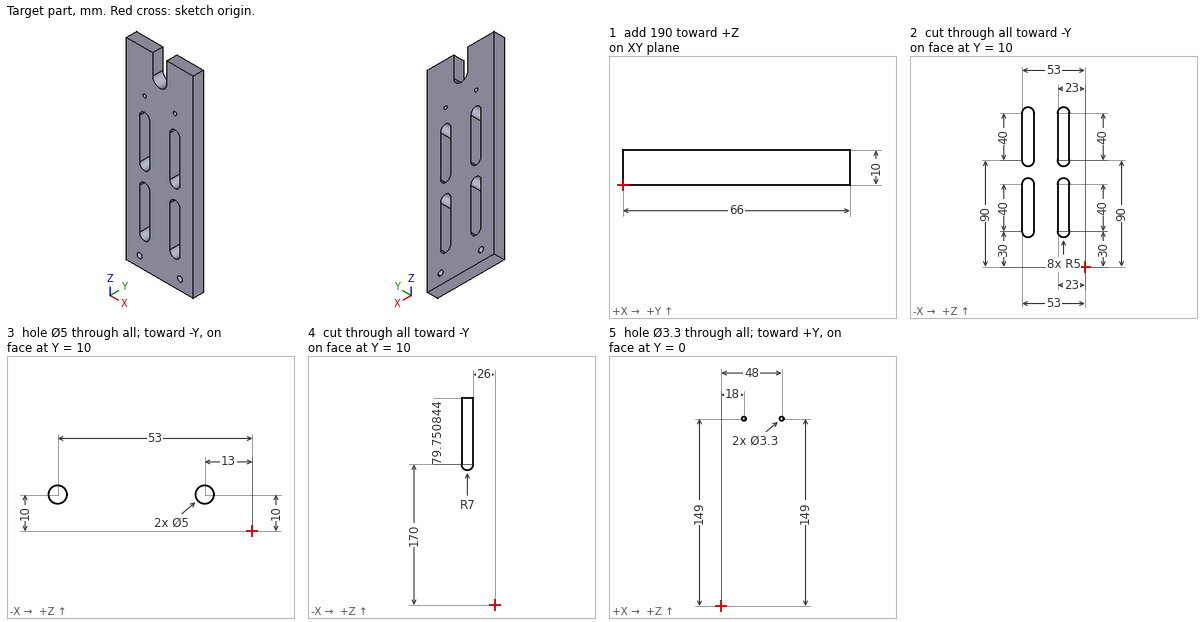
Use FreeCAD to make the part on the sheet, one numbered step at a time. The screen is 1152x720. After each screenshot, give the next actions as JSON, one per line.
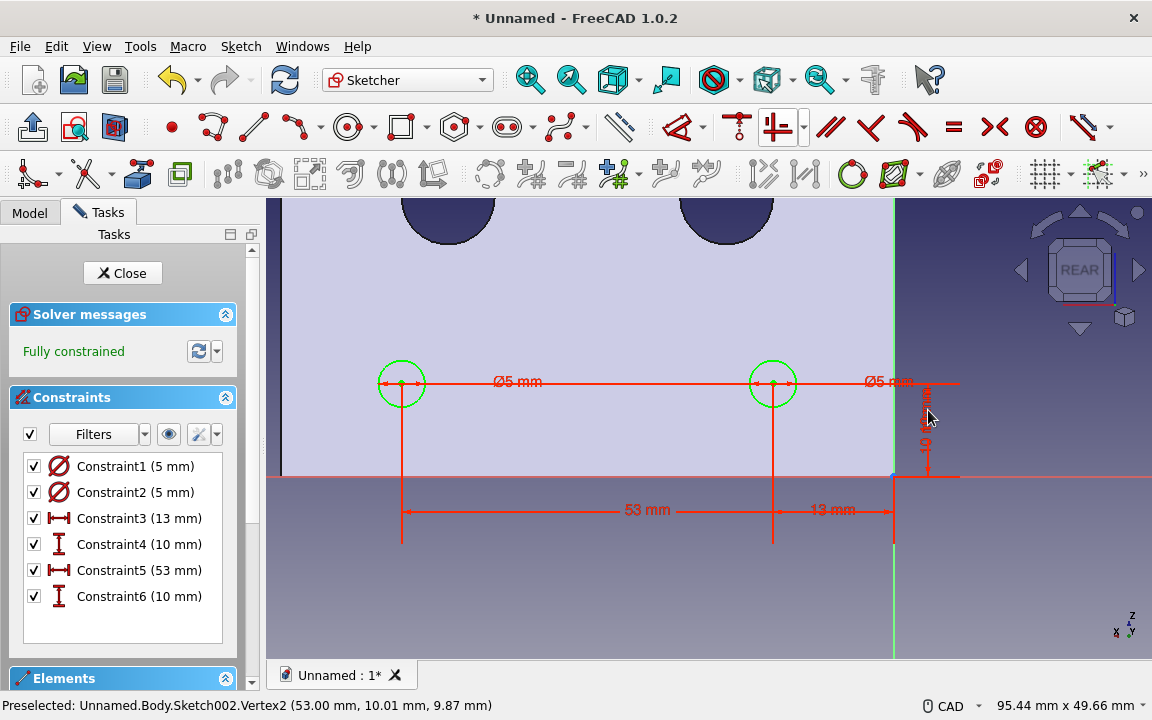
{"action": "left_click", "coordinate": [123, 273]}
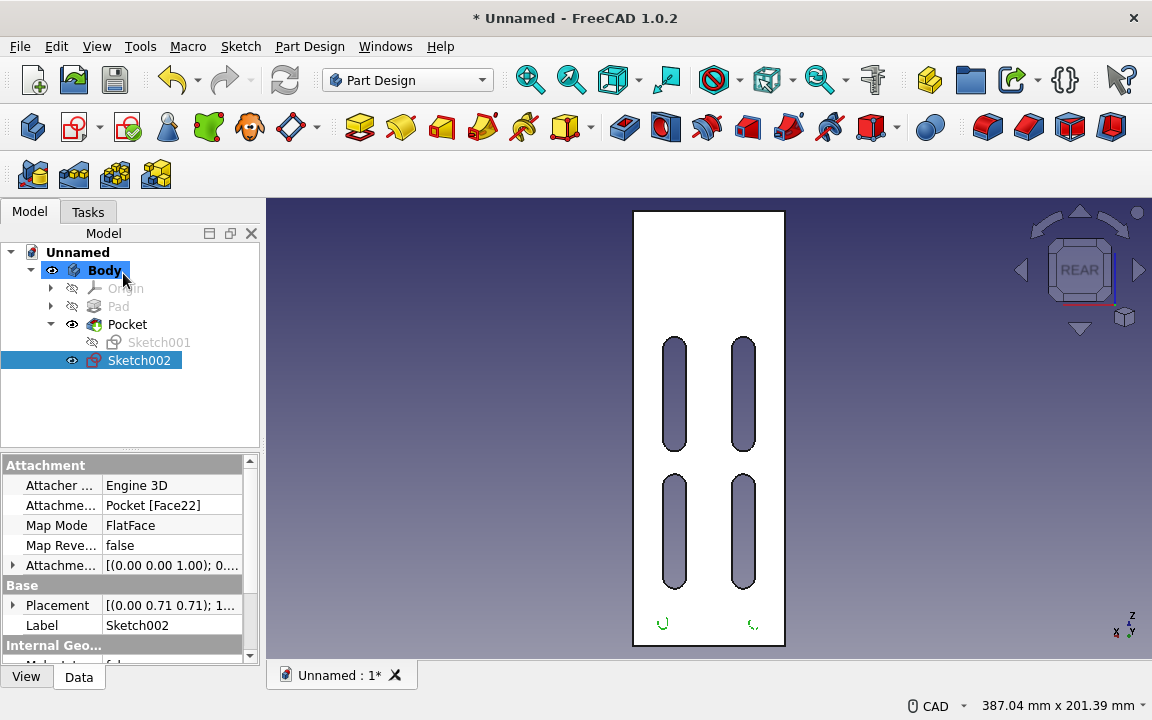
{"action": "left_click", "coordinate": [666, 128]}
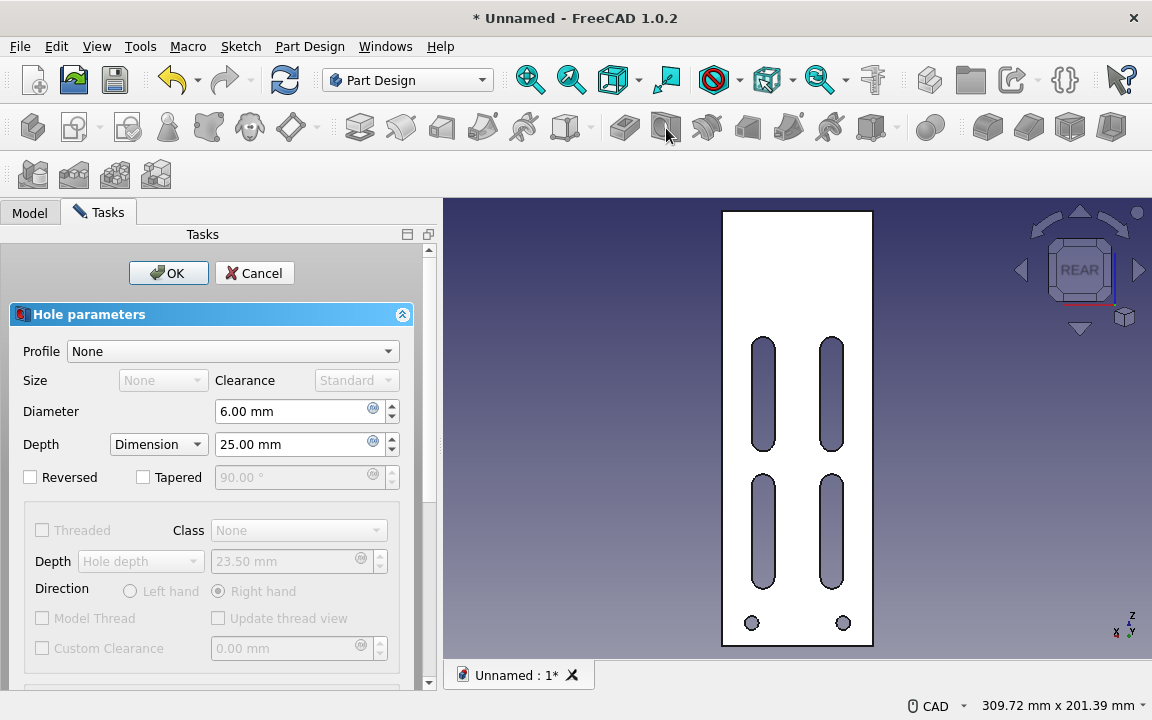
{"action": "triple_click", "coordinate": [300, 412]}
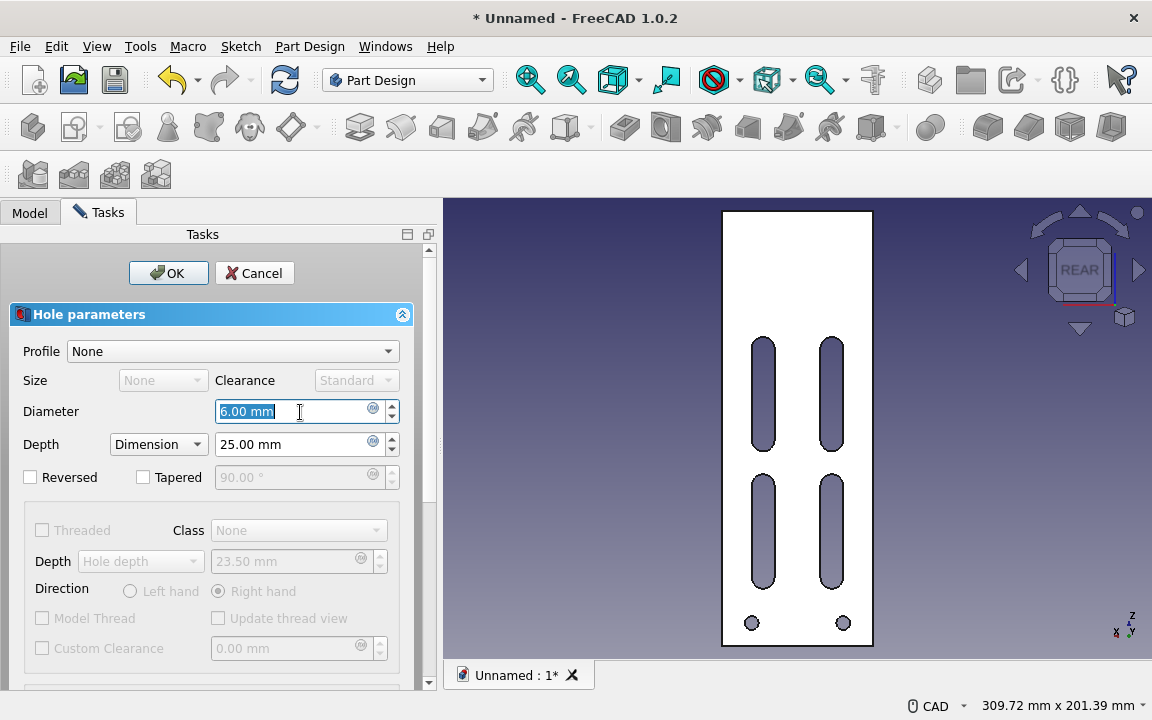
{"action": "type", "text": "5"}
{"action": "key", "text": "Tab"}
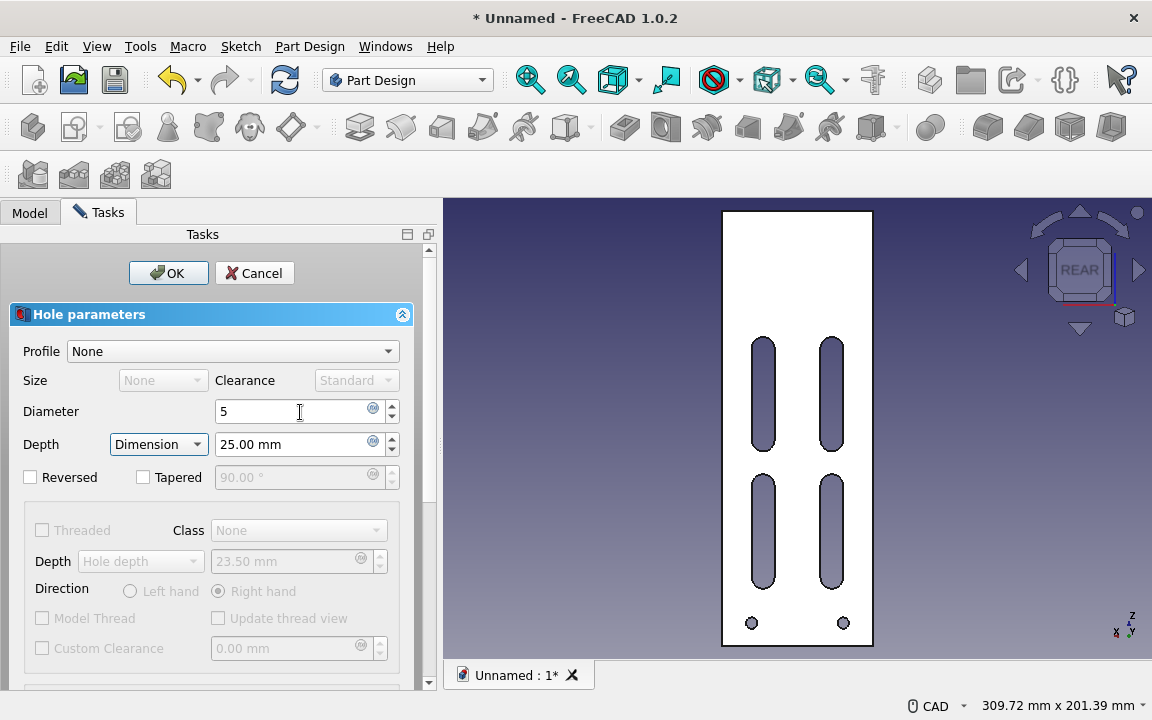
{"action": "left_click", "coordinate": [160, 444]}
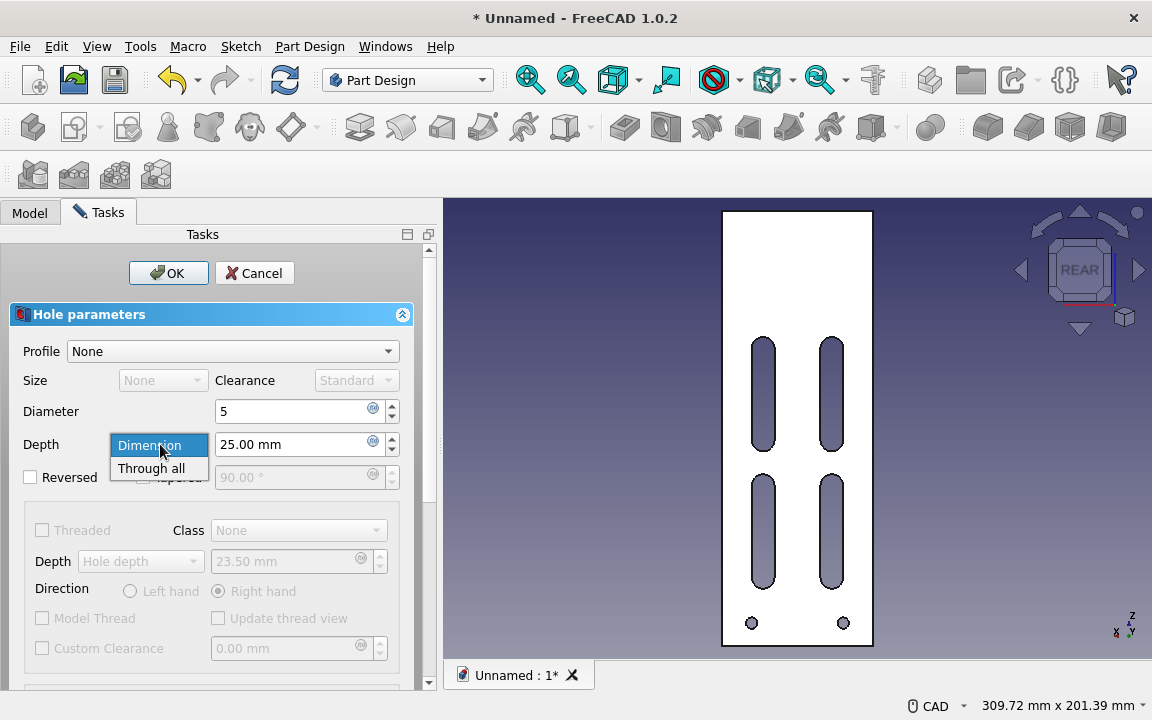
{"action": "left_click", "coordinate": [158, 468]}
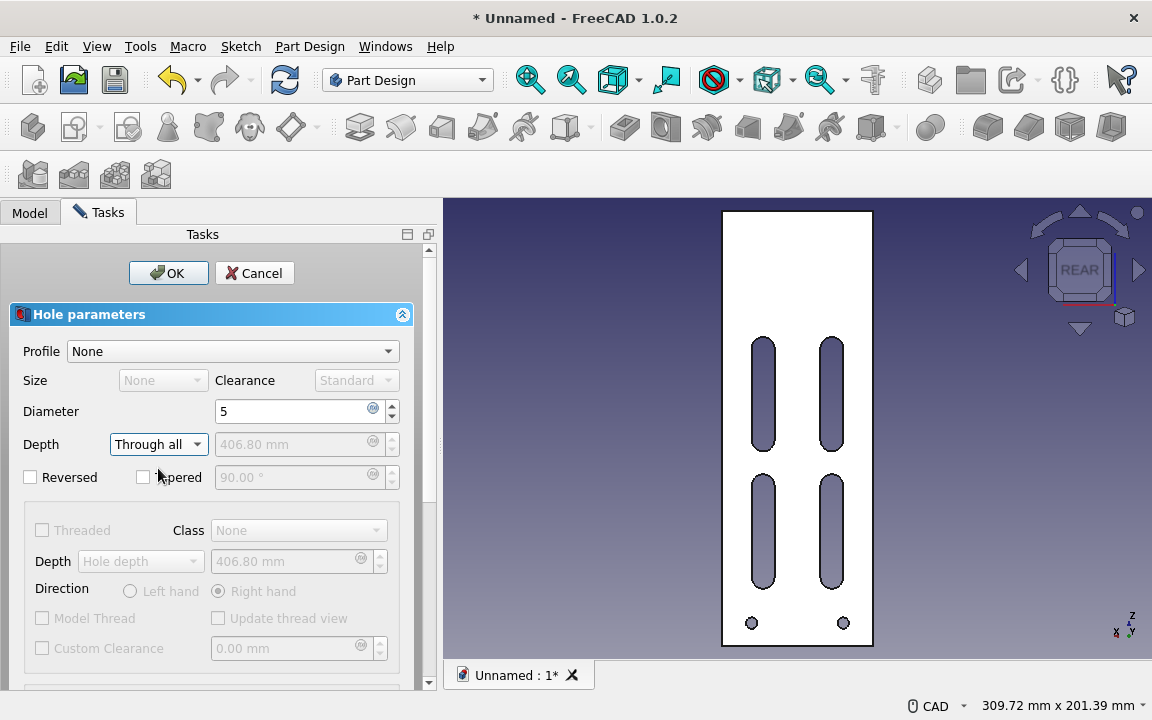
{"action": "left_click", "coordinate": [169, 273]}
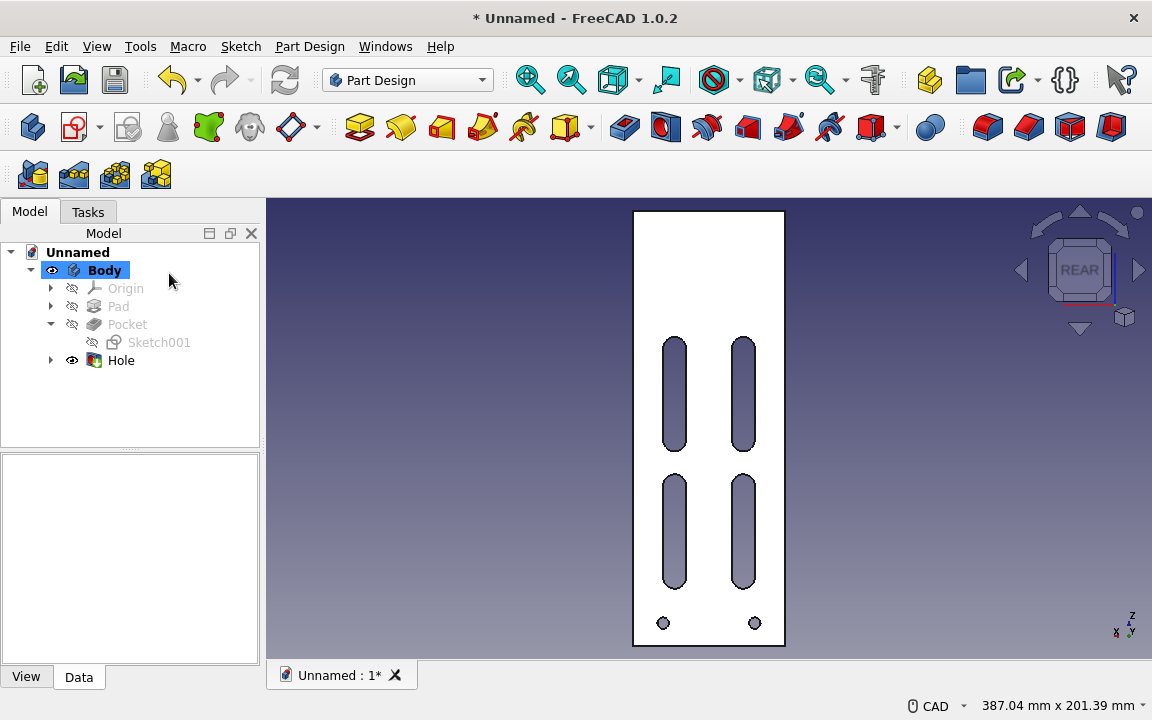
{"action": "left_click", "coordinate": [709, 303]}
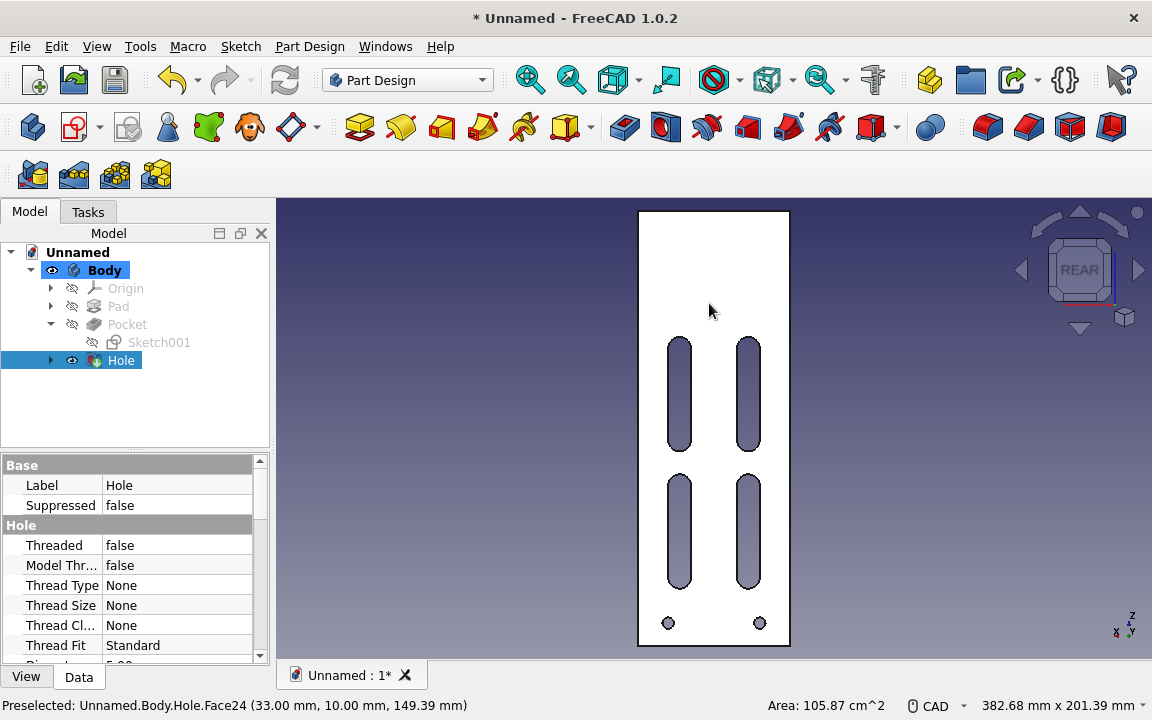
{"action": "left_click", "coordinate": [74, 128]}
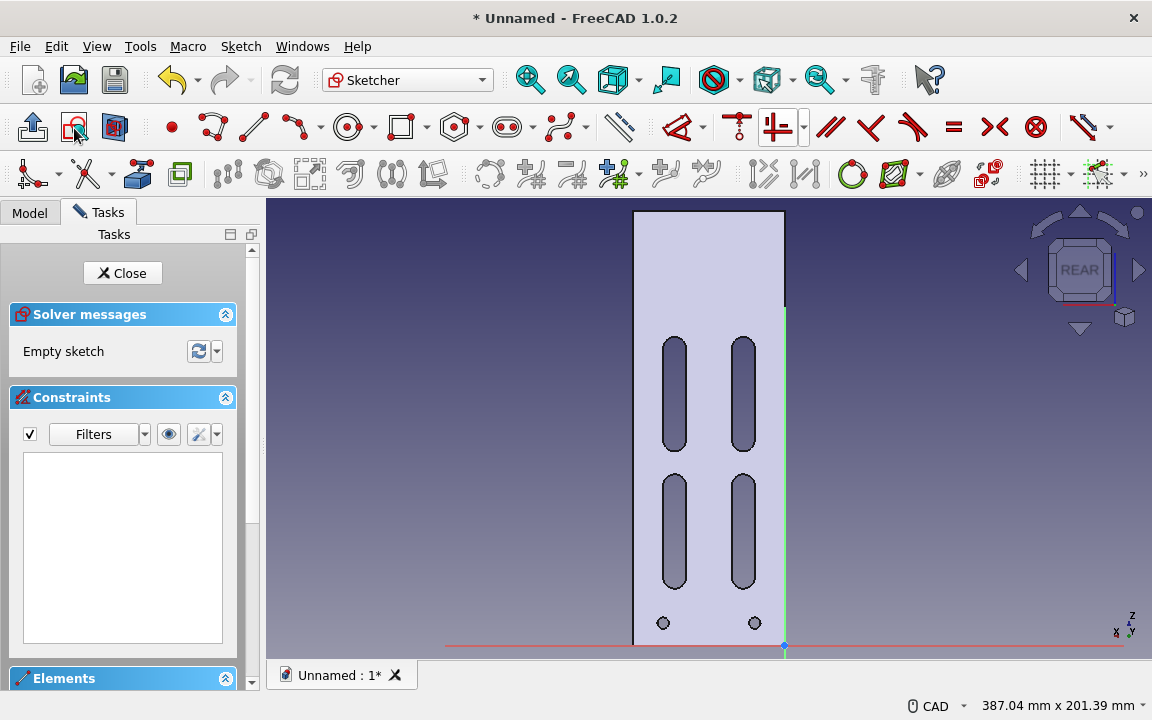
{"action": "scroll", "coordinate": [640, 428], "scroll_direction": "down", "scroll_amount": 5}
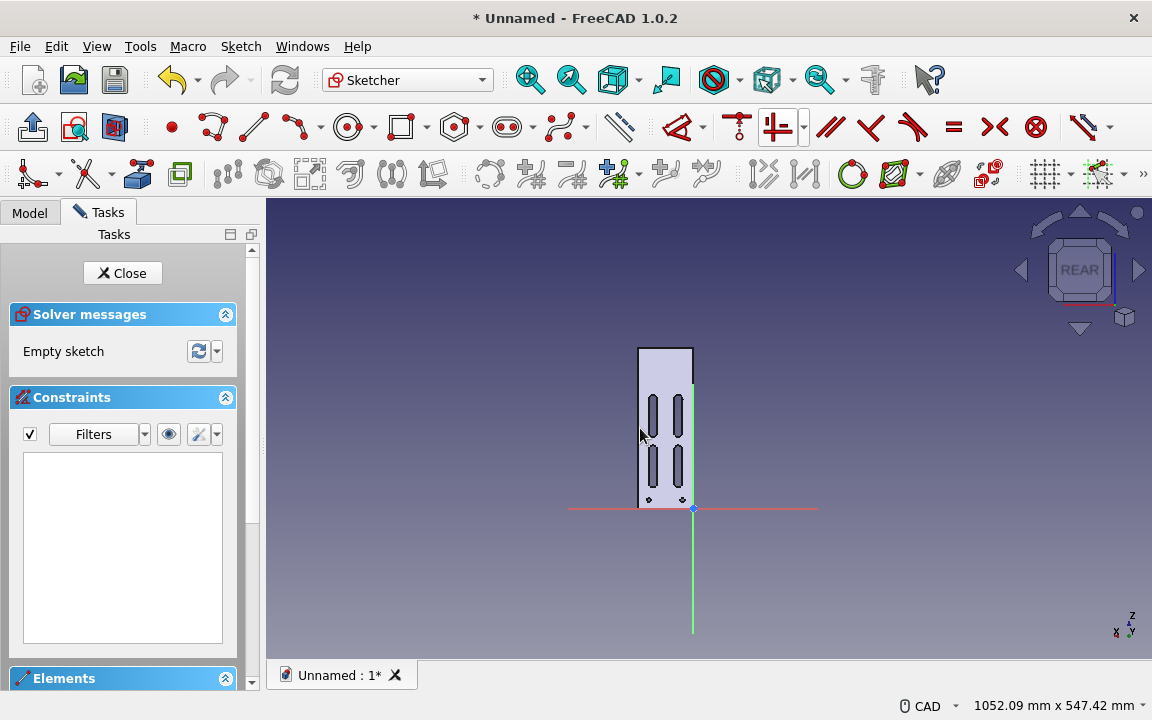
{"action": "scroll", "coordinate": [674, 304], "scroll_direction": "up", "scroll_amount": 7}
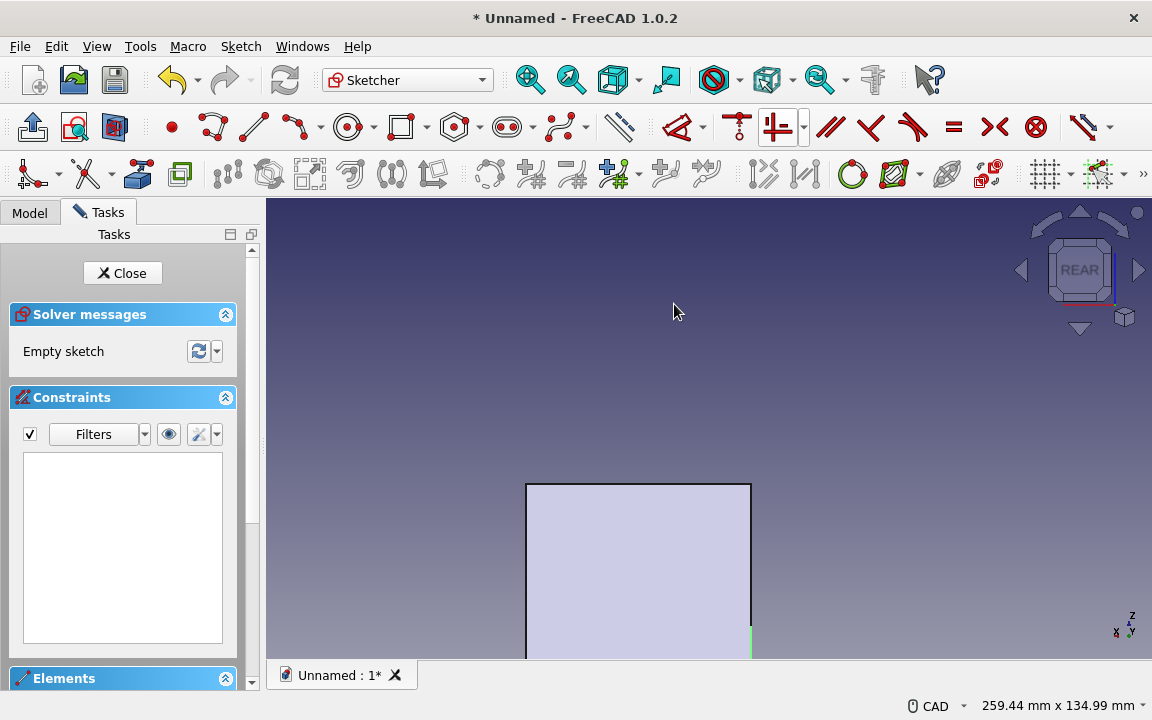
{"action": "left_click", "coordinate": [213, 128]}